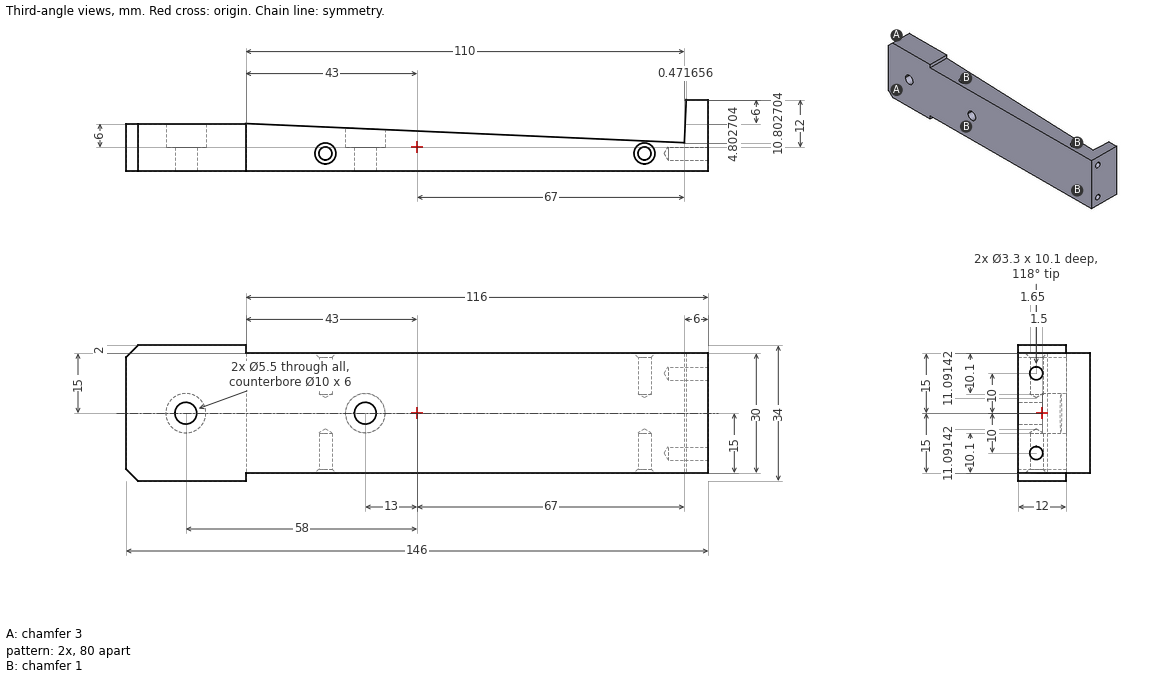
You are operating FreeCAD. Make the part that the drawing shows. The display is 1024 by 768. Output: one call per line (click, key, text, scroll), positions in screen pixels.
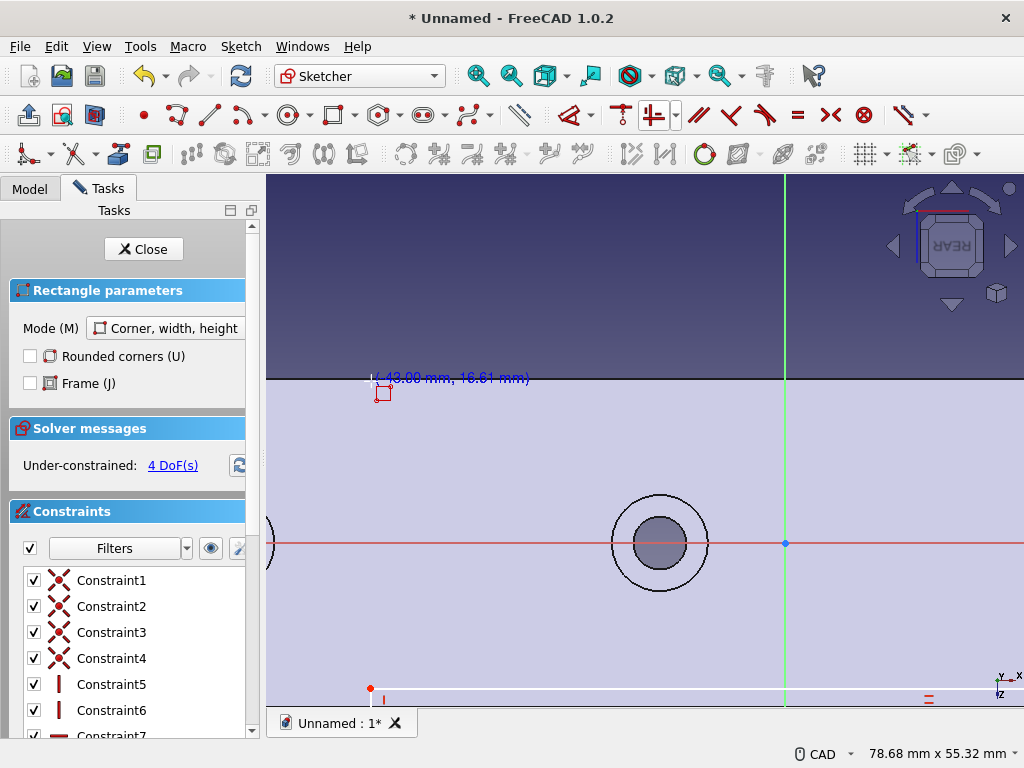
click(371, 379)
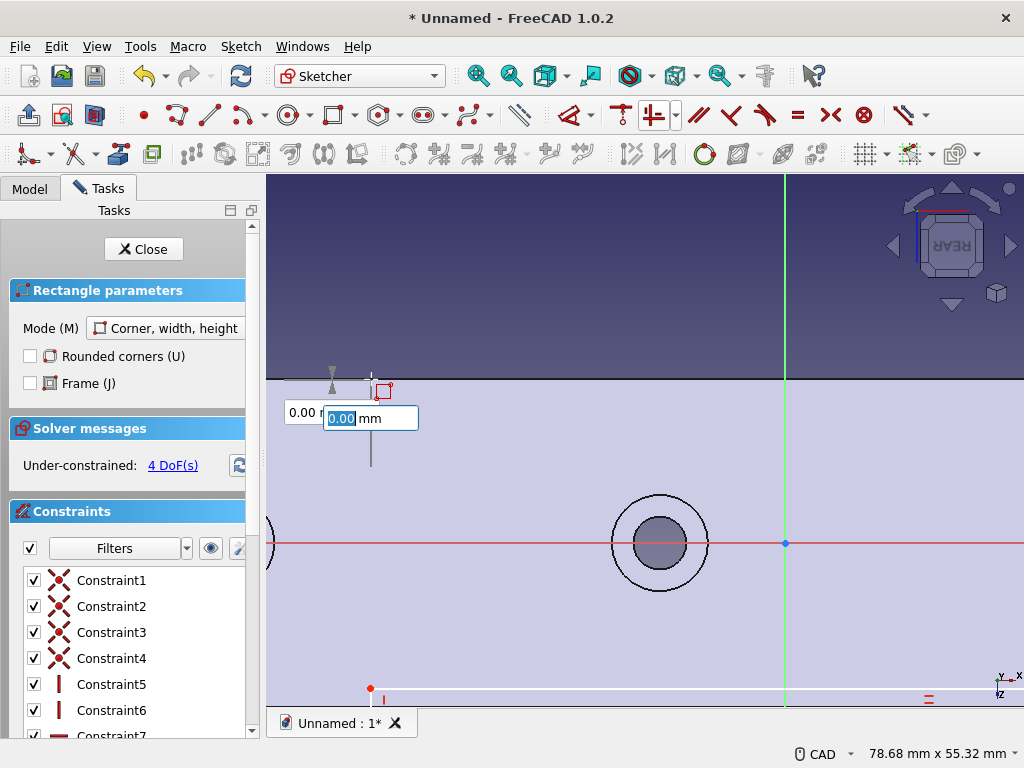
scroll(371, 381, down, 5)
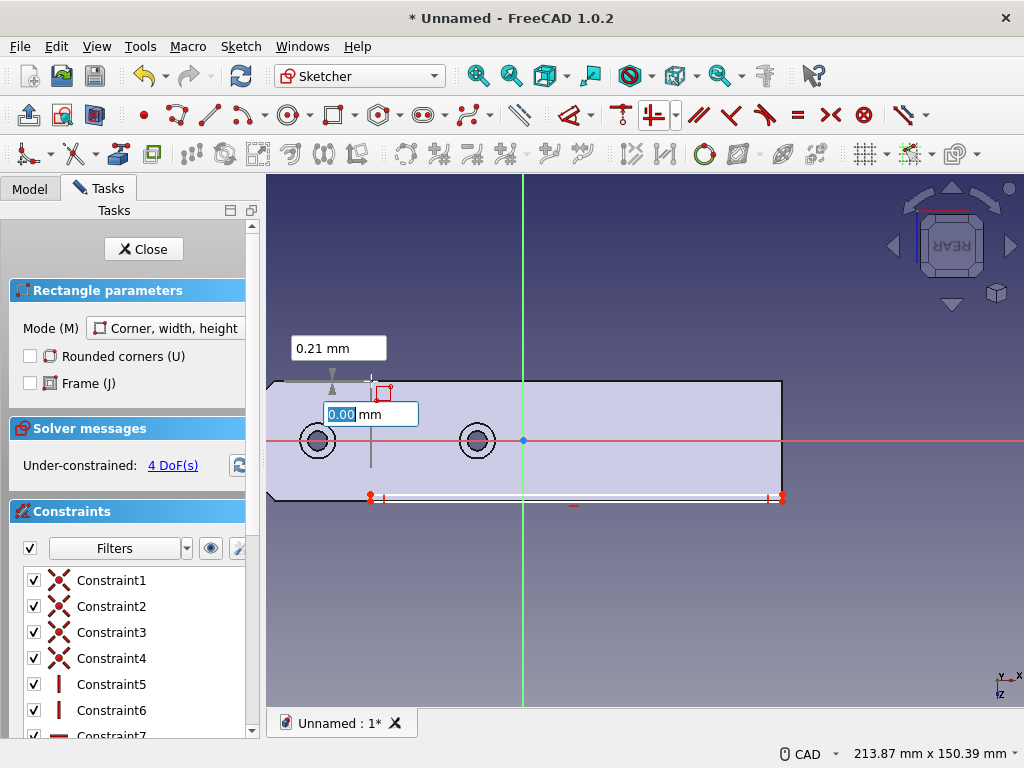
click(782, 388)
key(Escape)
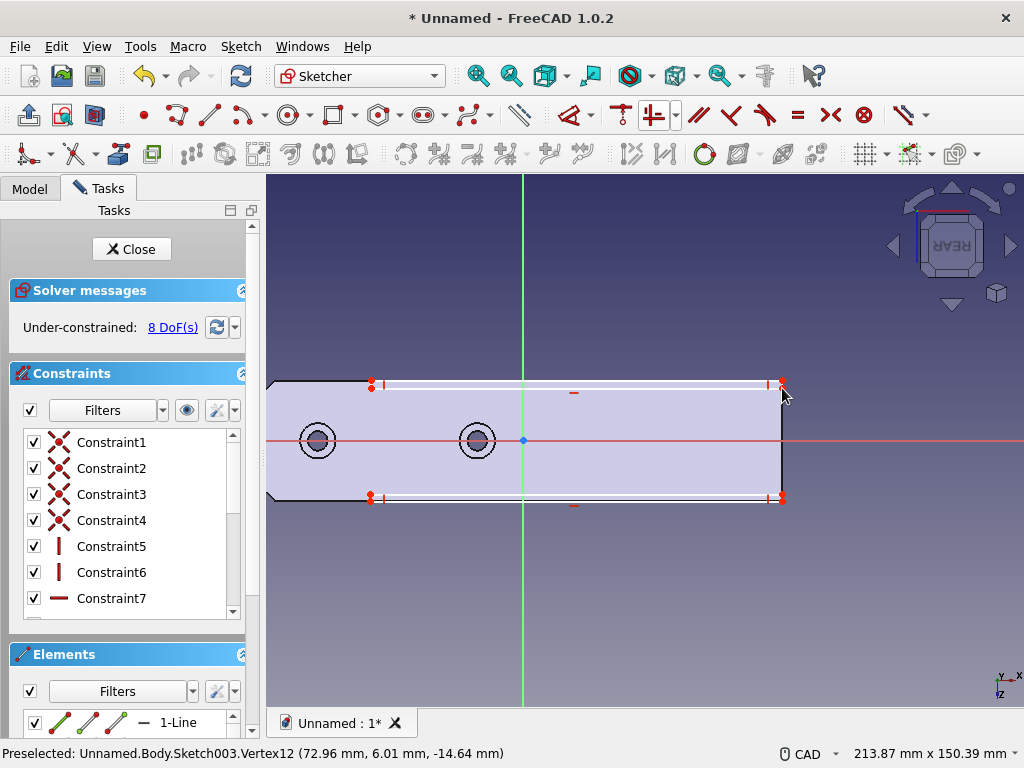
scroll(371, 502, up, 3)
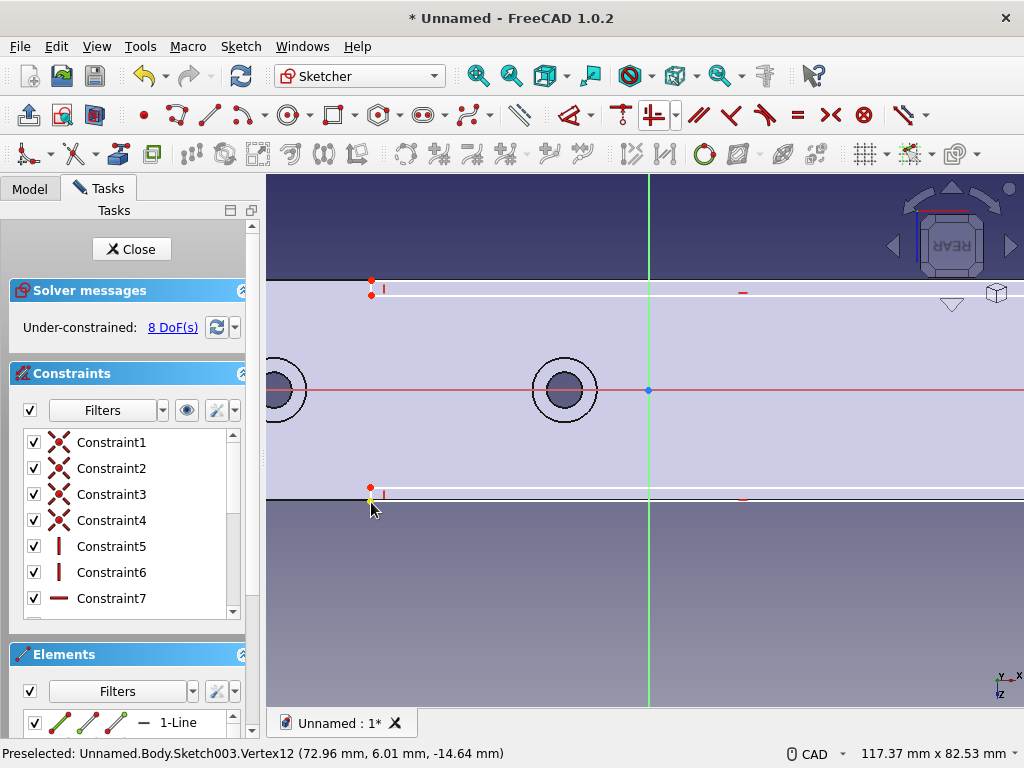
click(371, 501)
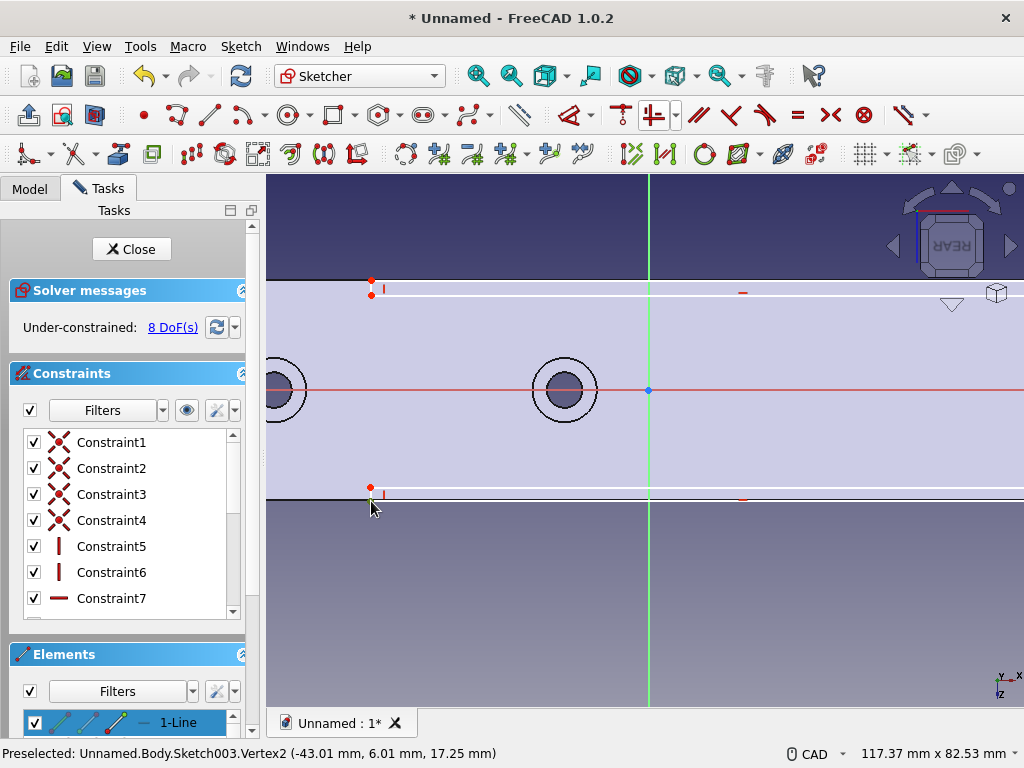
click(371, 281)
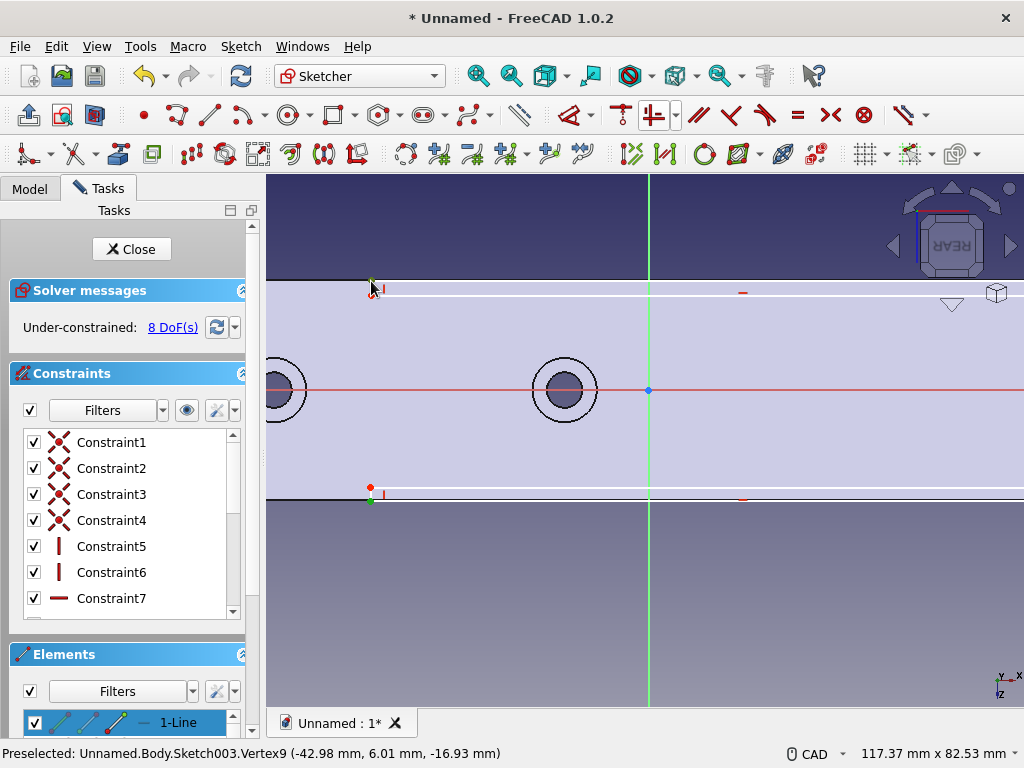
click(334, 390)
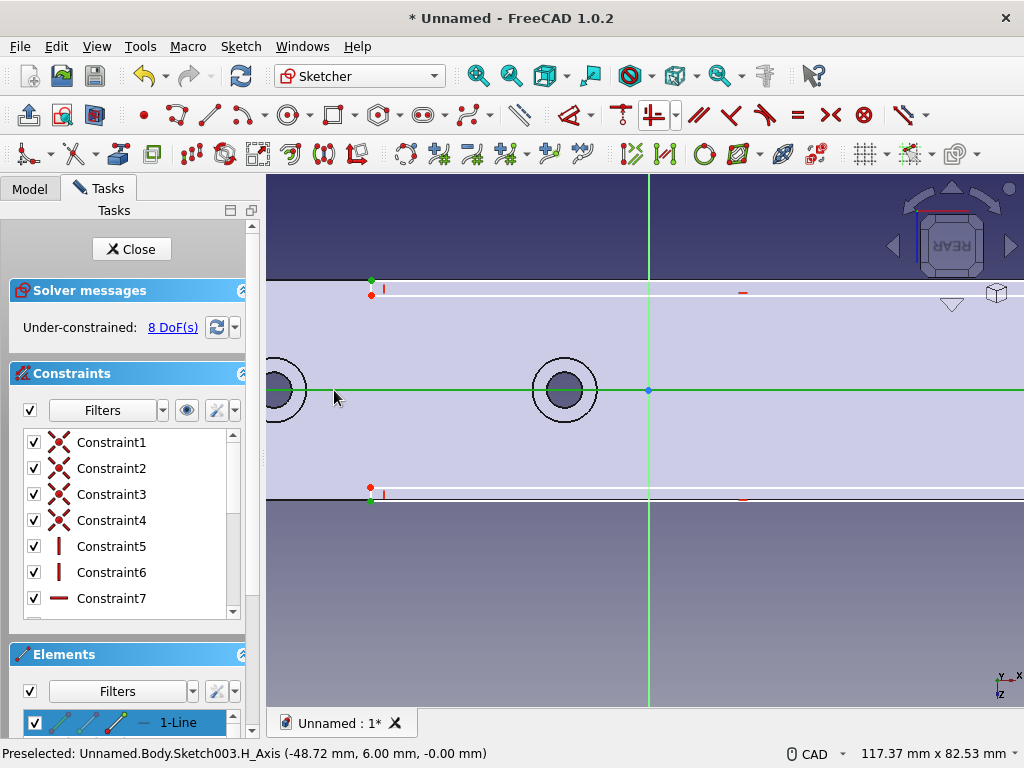
key(s)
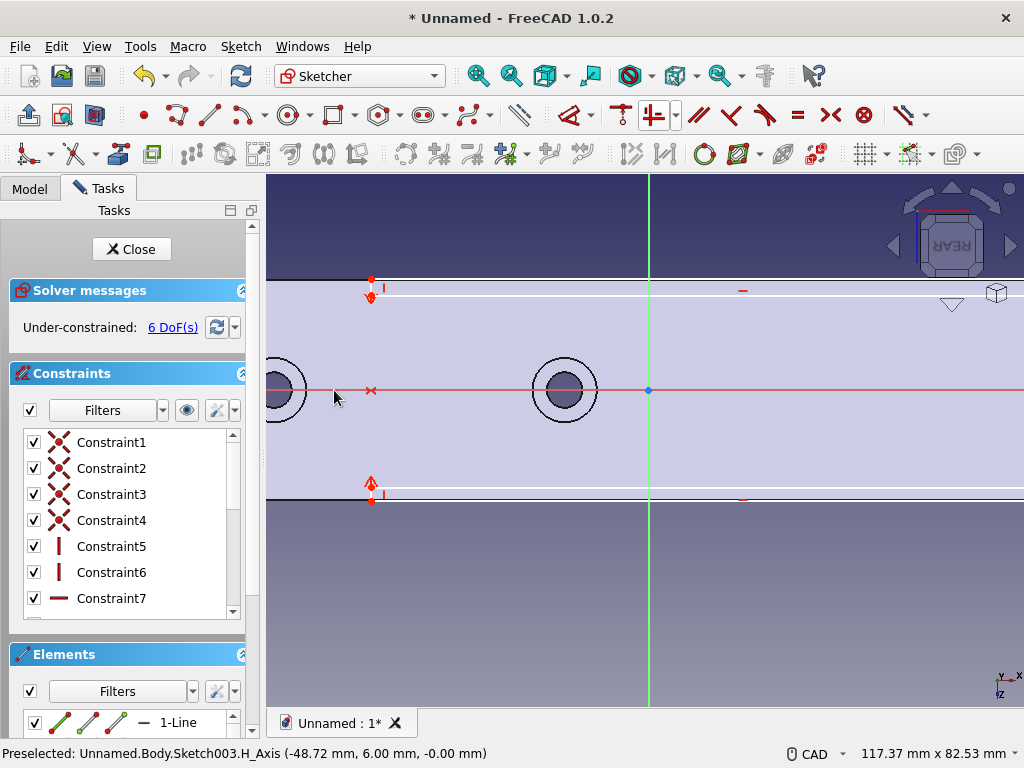
scroll(371, 502, down, 3)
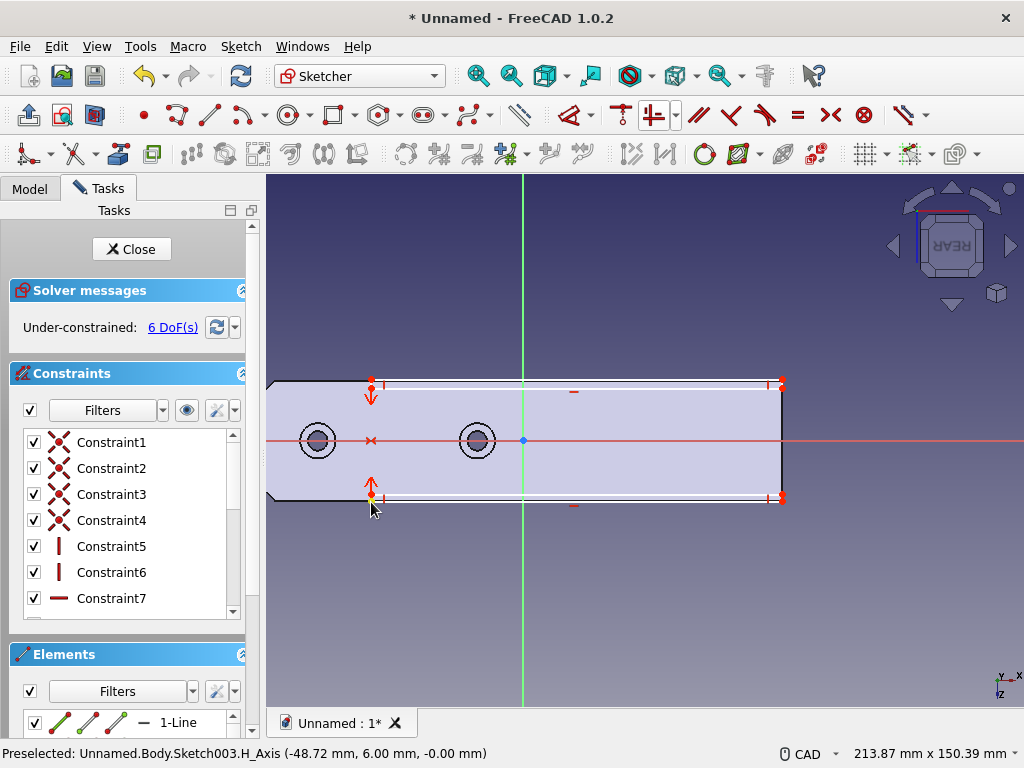
scroll(782, 495, up, 3)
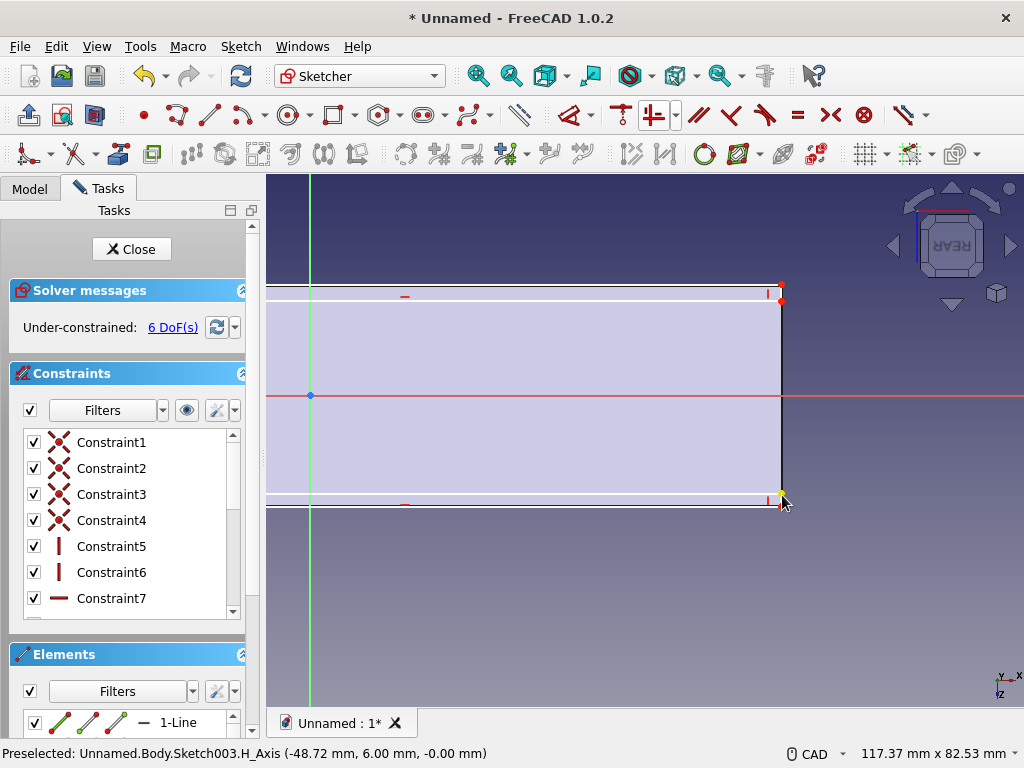
click(781, 494)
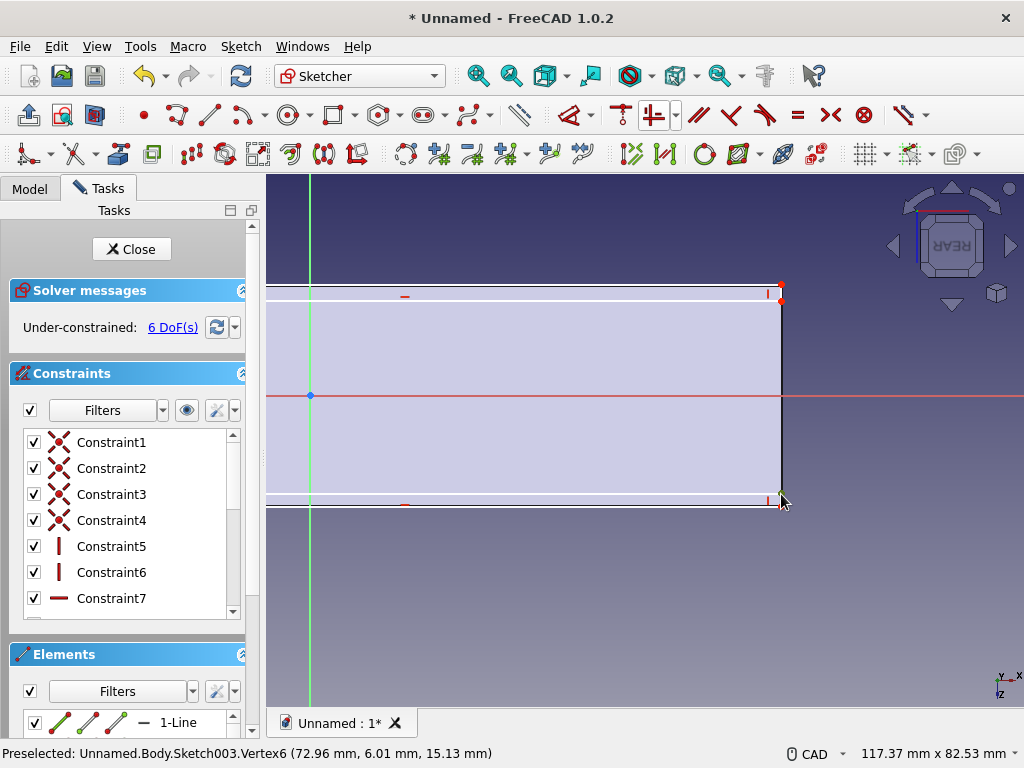
click(781, 301)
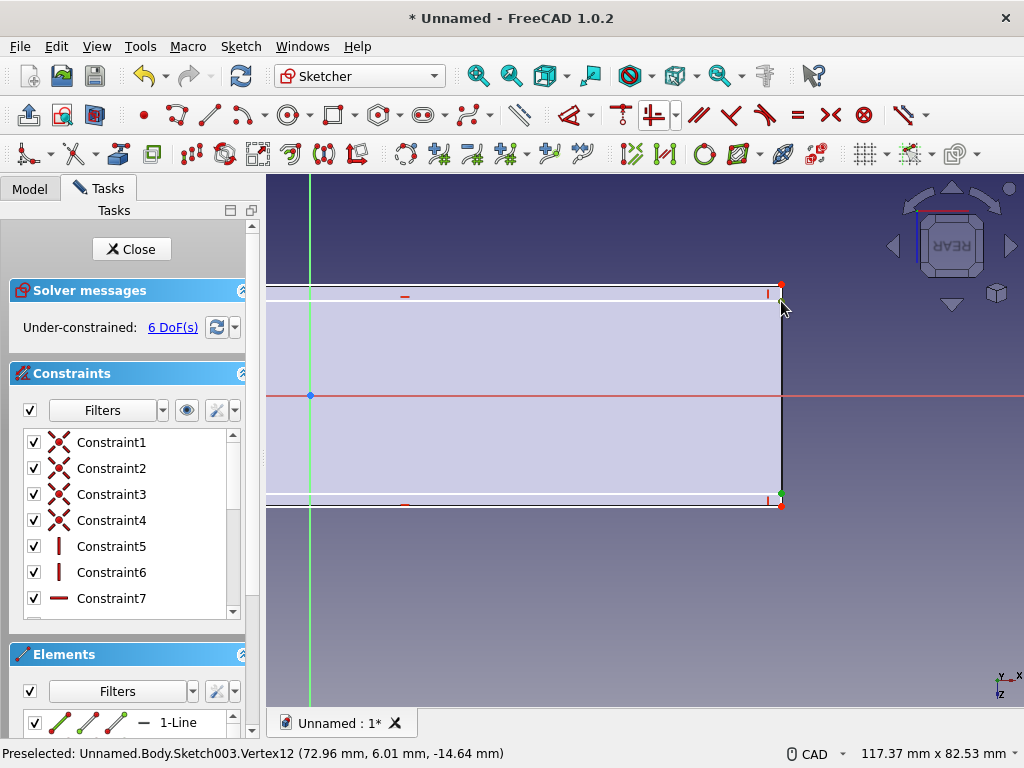
click(375, 396)